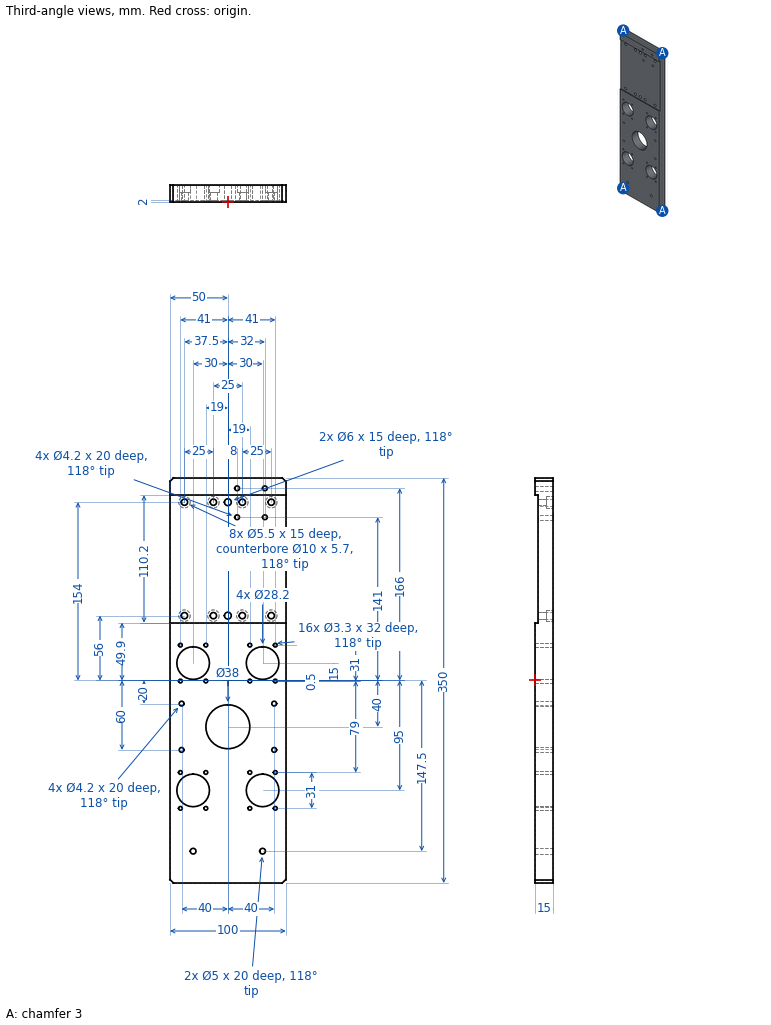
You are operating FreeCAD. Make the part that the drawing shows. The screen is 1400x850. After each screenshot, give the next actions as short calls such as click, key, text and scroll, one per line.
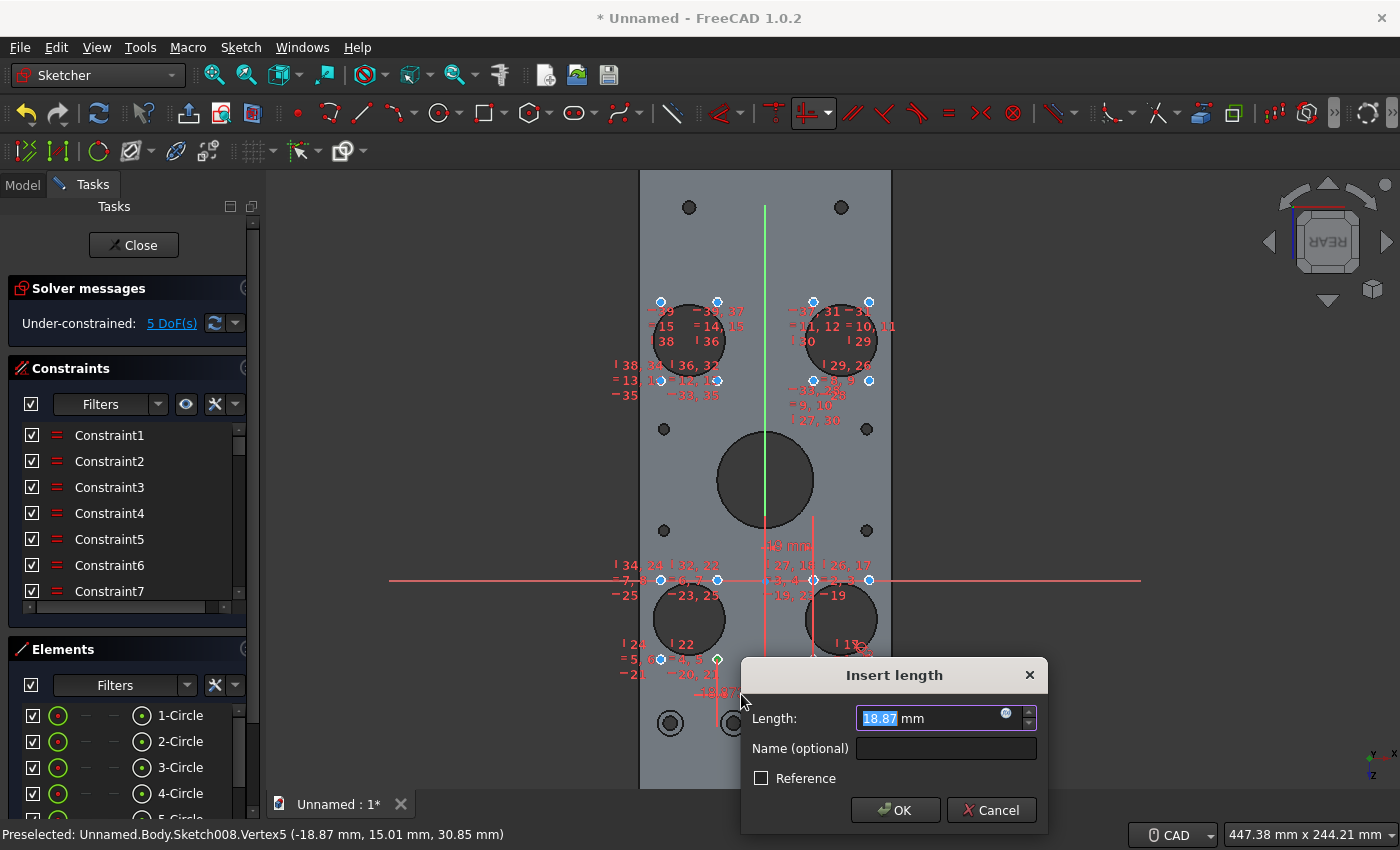
text(19)
key(Return)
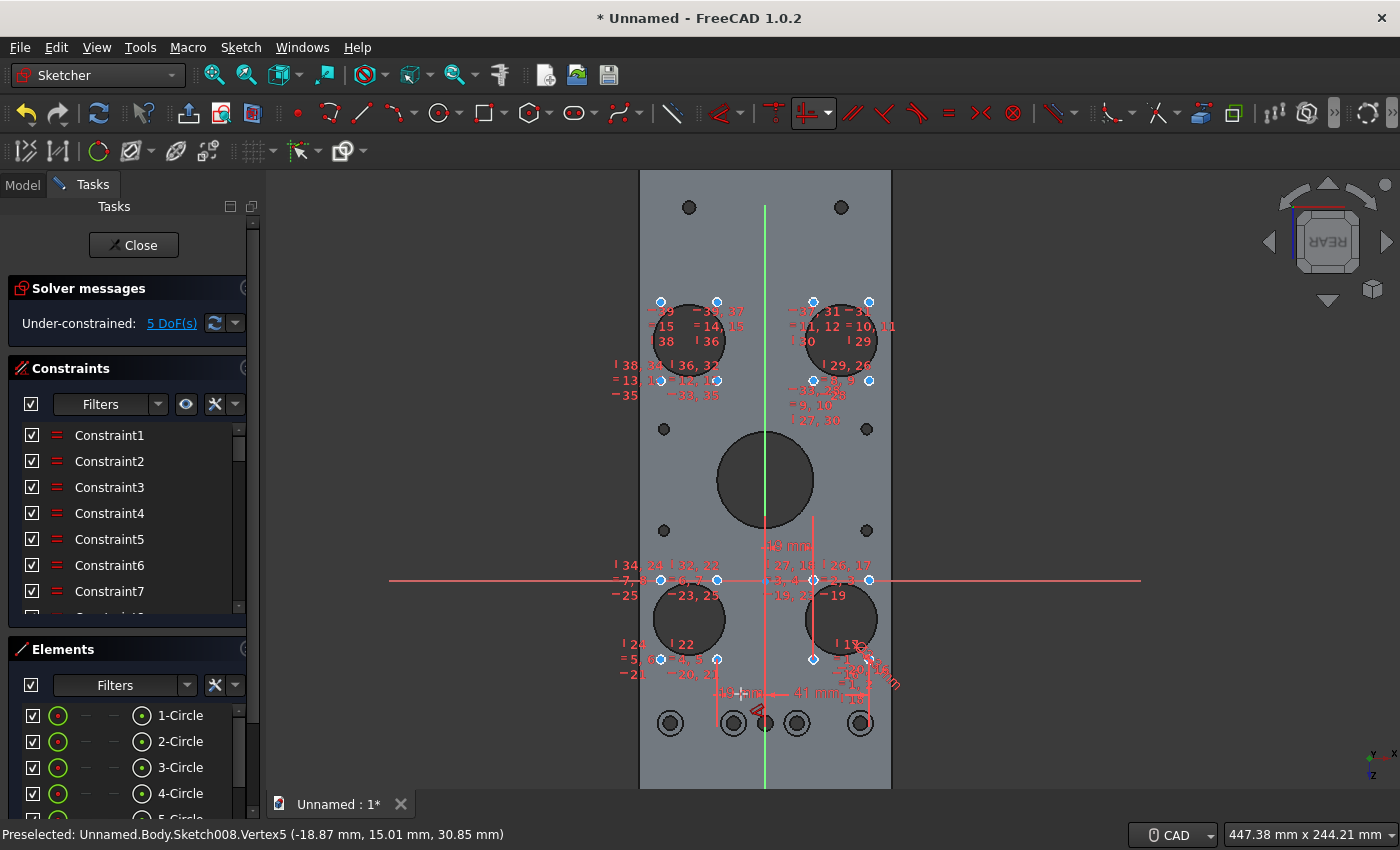
click(661, 660)
click(713, 547)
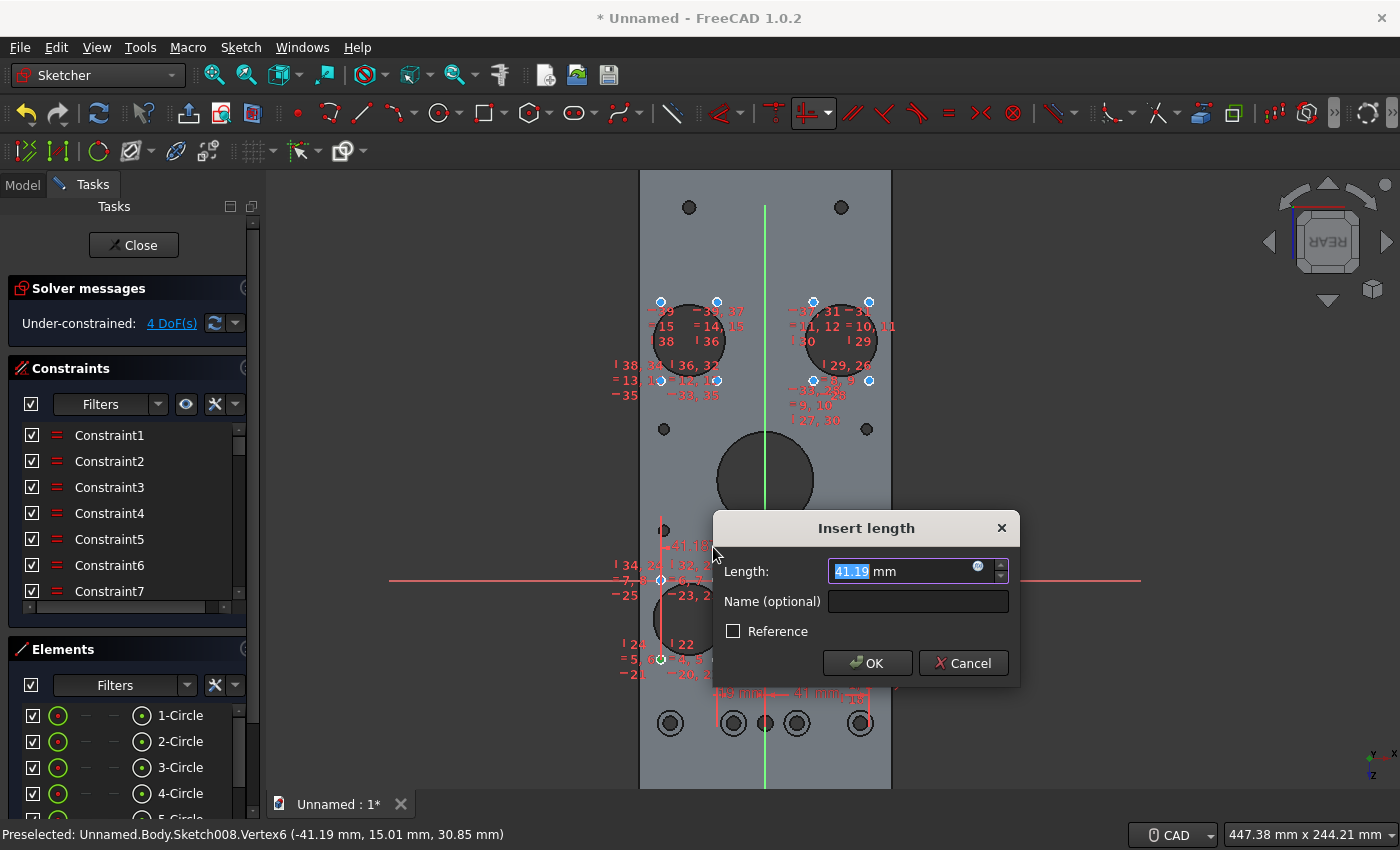
text(41)
key(Return)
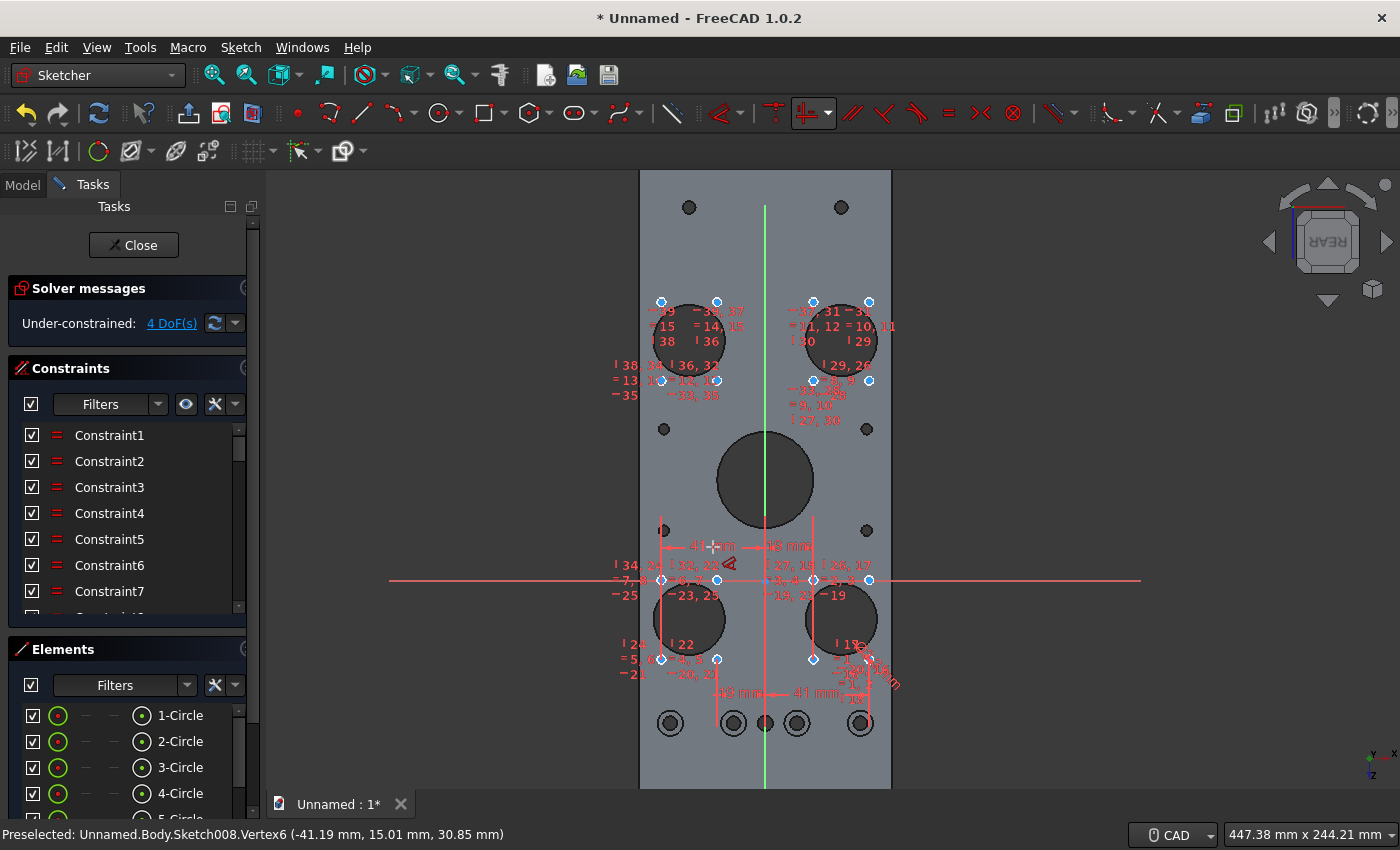
scroll(869, 580, up, 18)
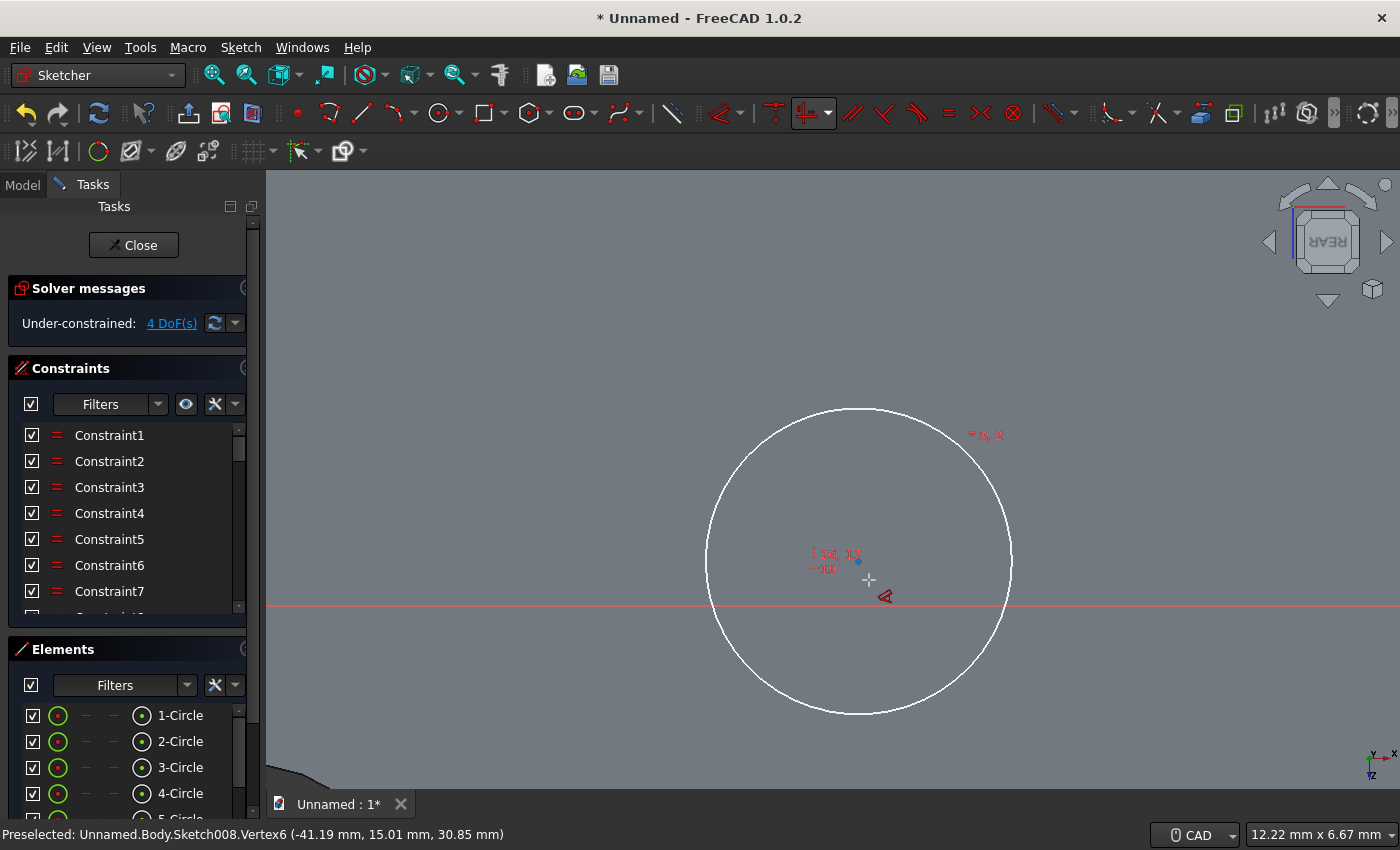
click(859, 561)
click(893, 584)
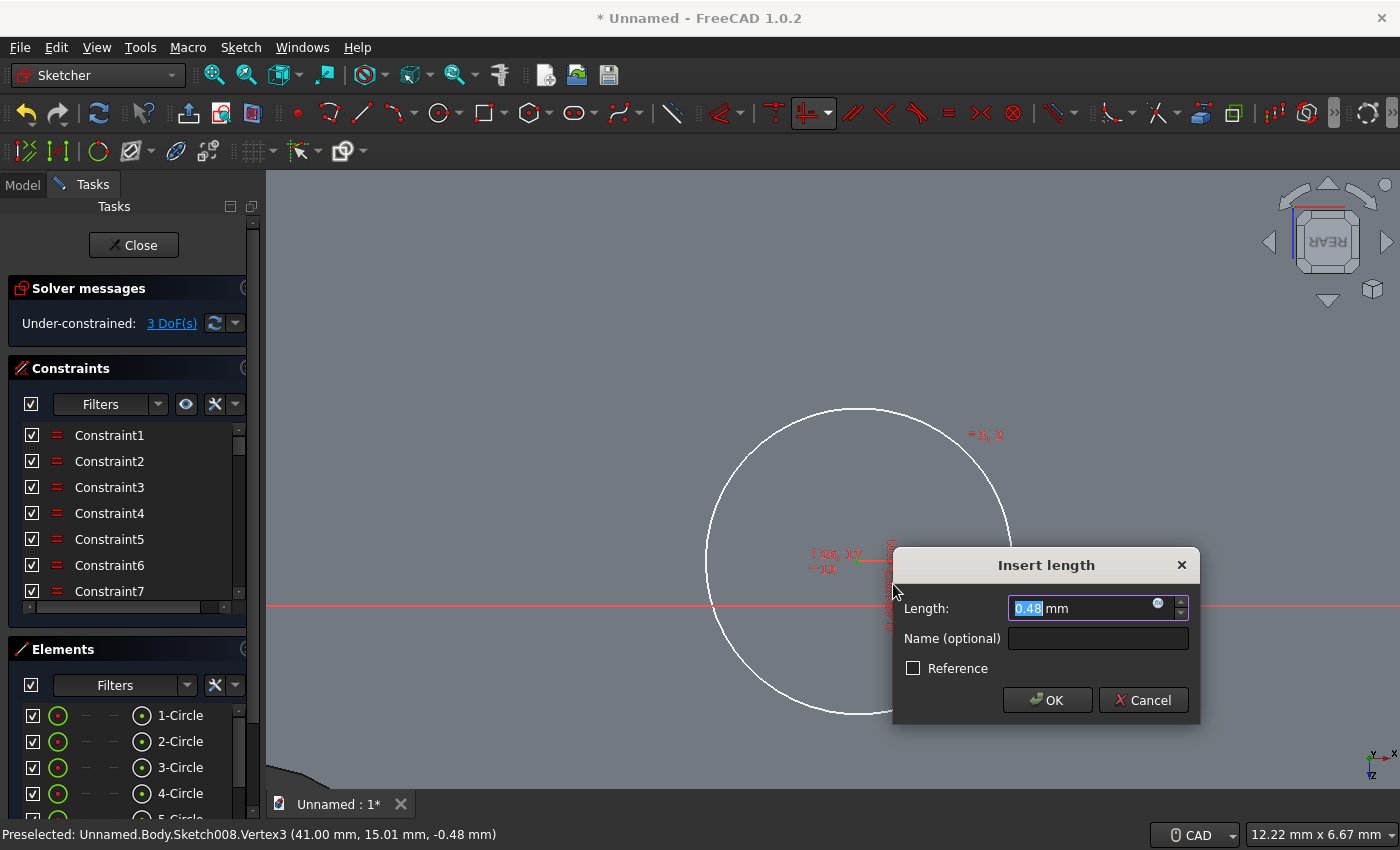
text(0.5)
key(Return)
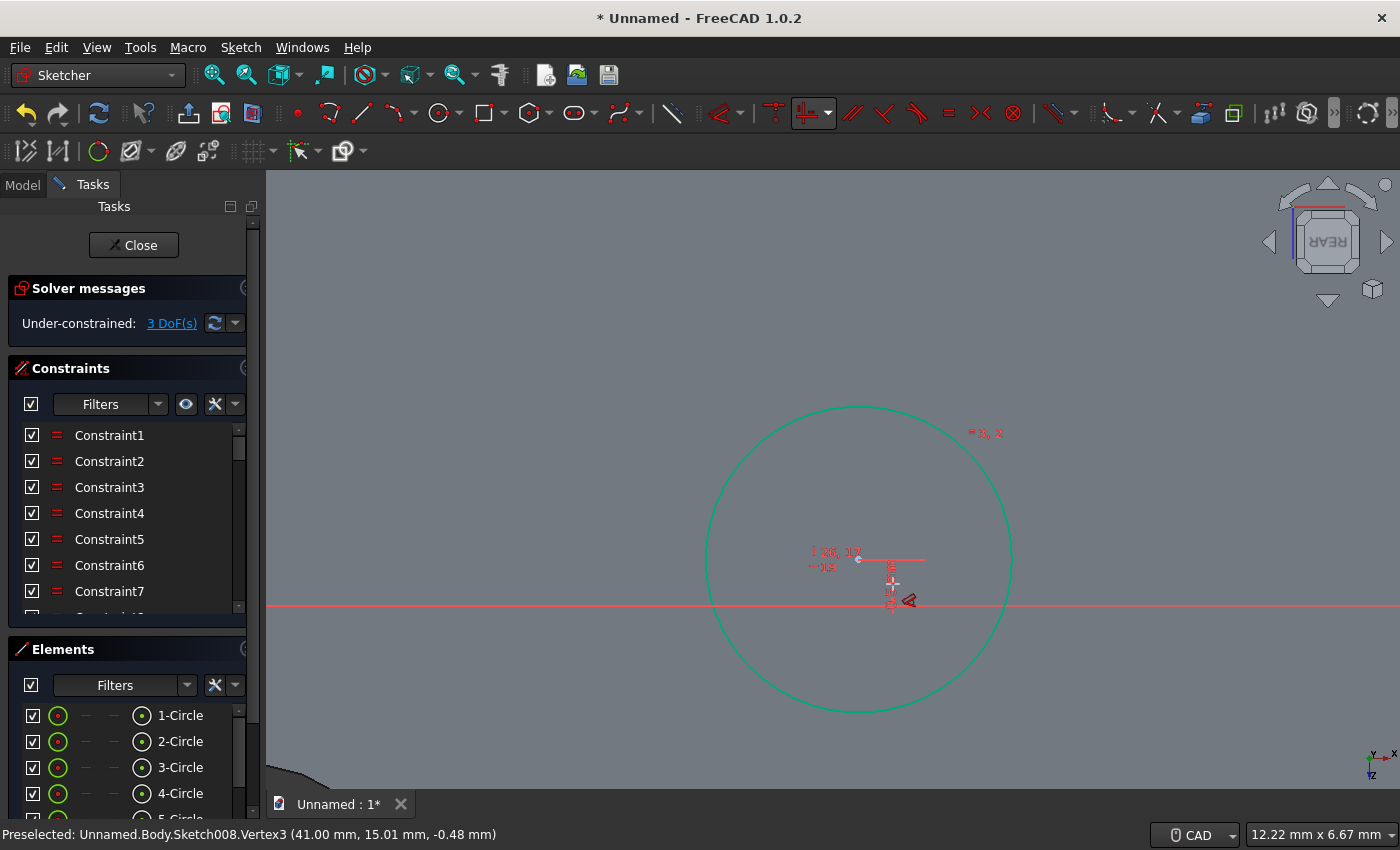
scroll(893, 603, down, 17)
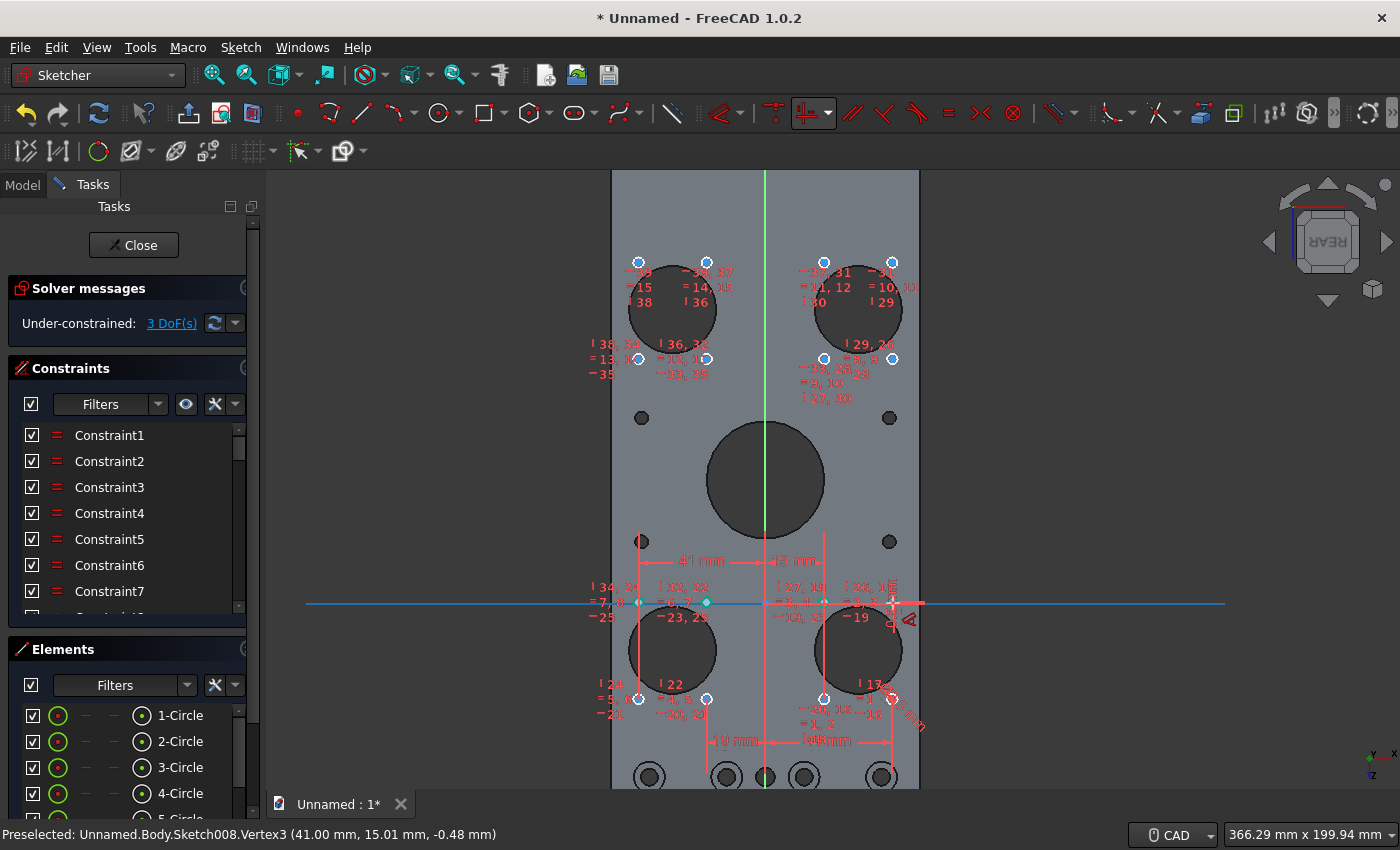
click(892, 699)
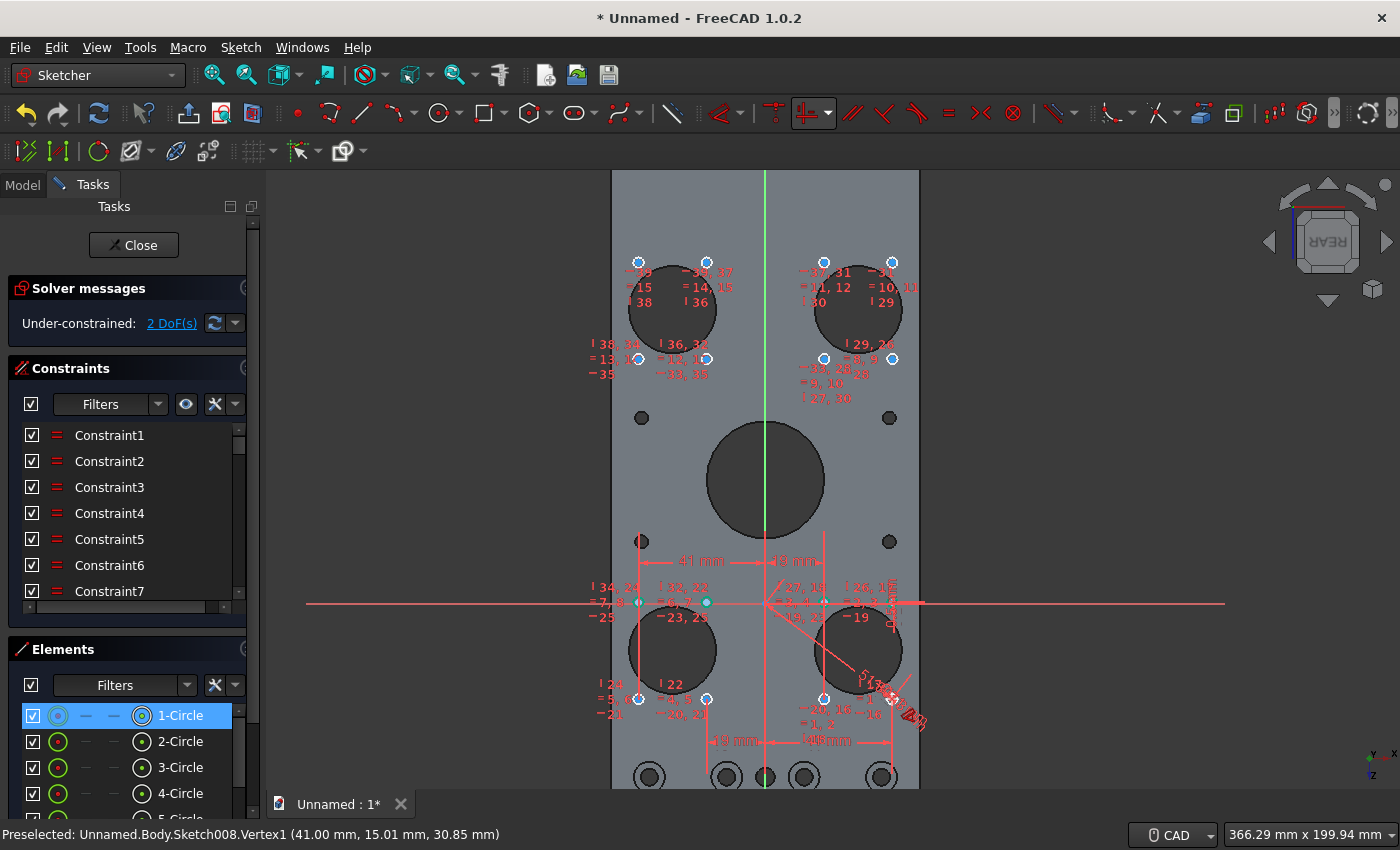
click(892, 602)
click(926, 651)